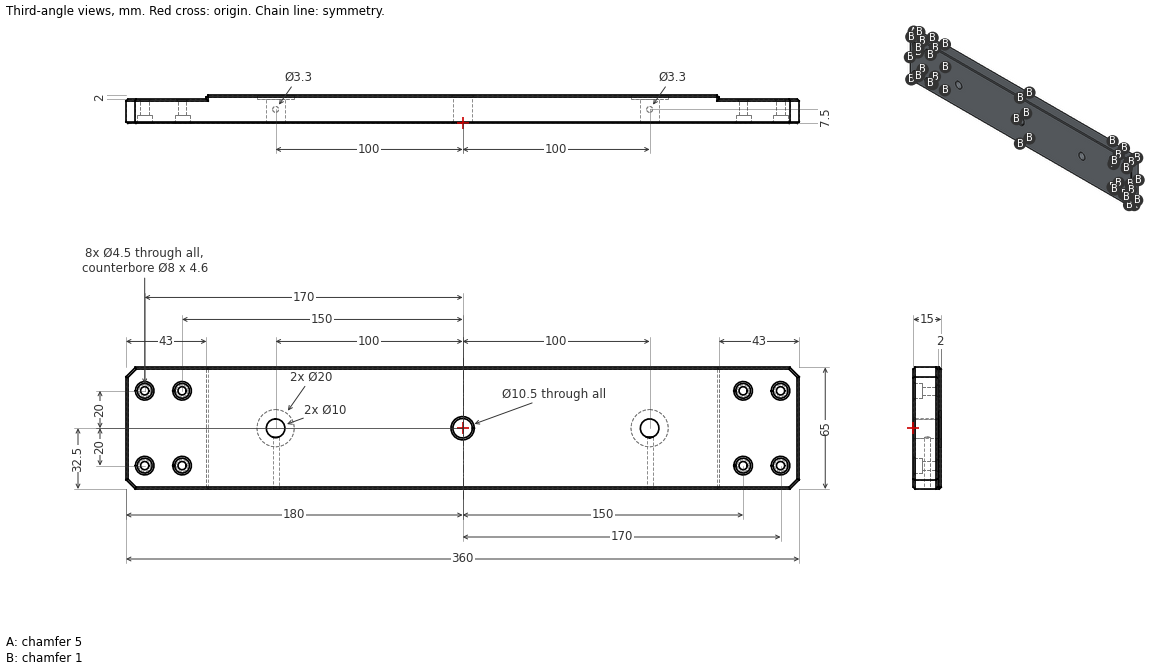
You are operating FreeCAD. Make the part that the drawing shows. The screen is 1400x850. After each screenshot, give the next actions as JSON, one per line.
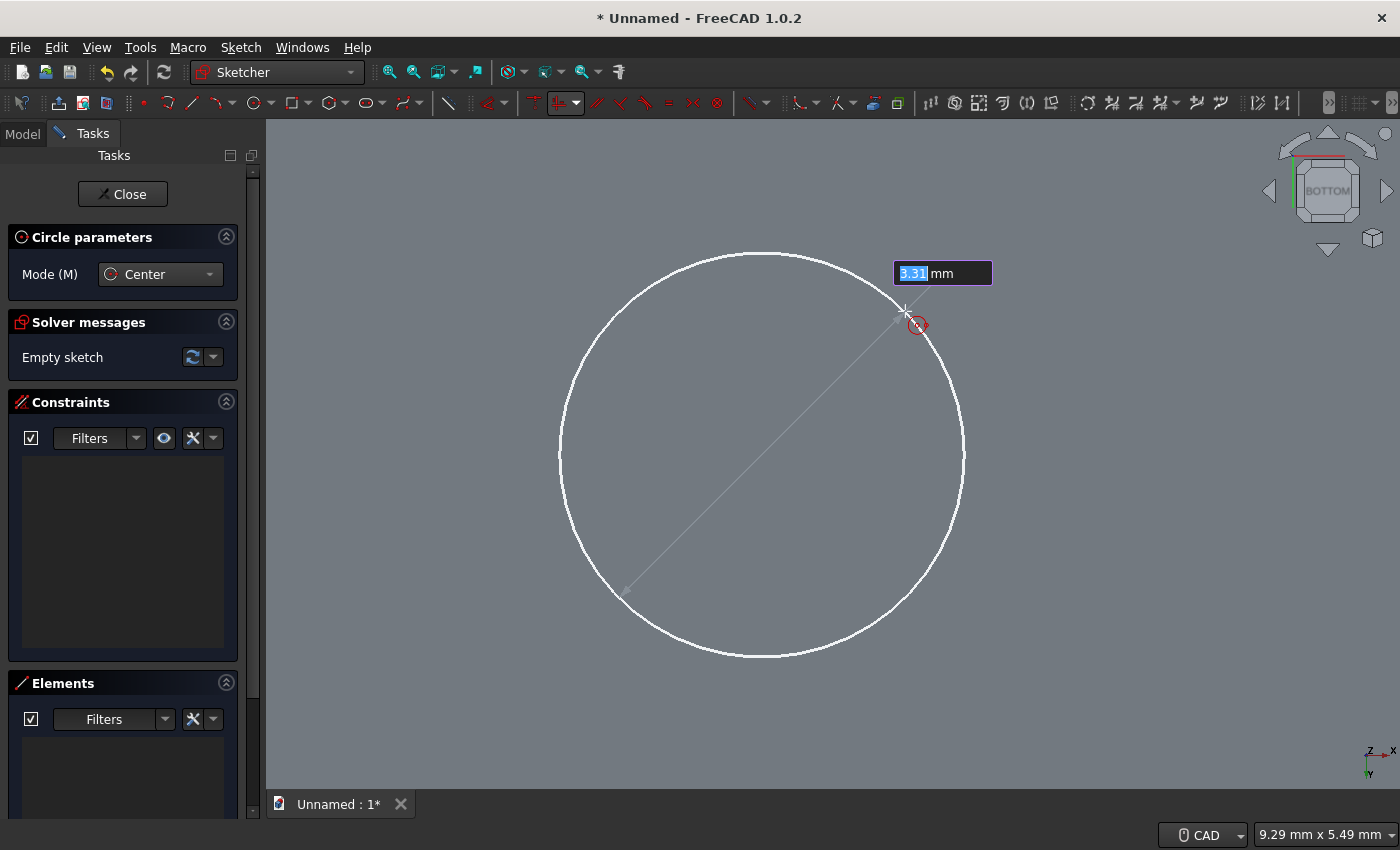
{"action": "type", "text": "3.3"}
{"action": "key", "text": "Return"}
{"action": "key", "text": "Escape"}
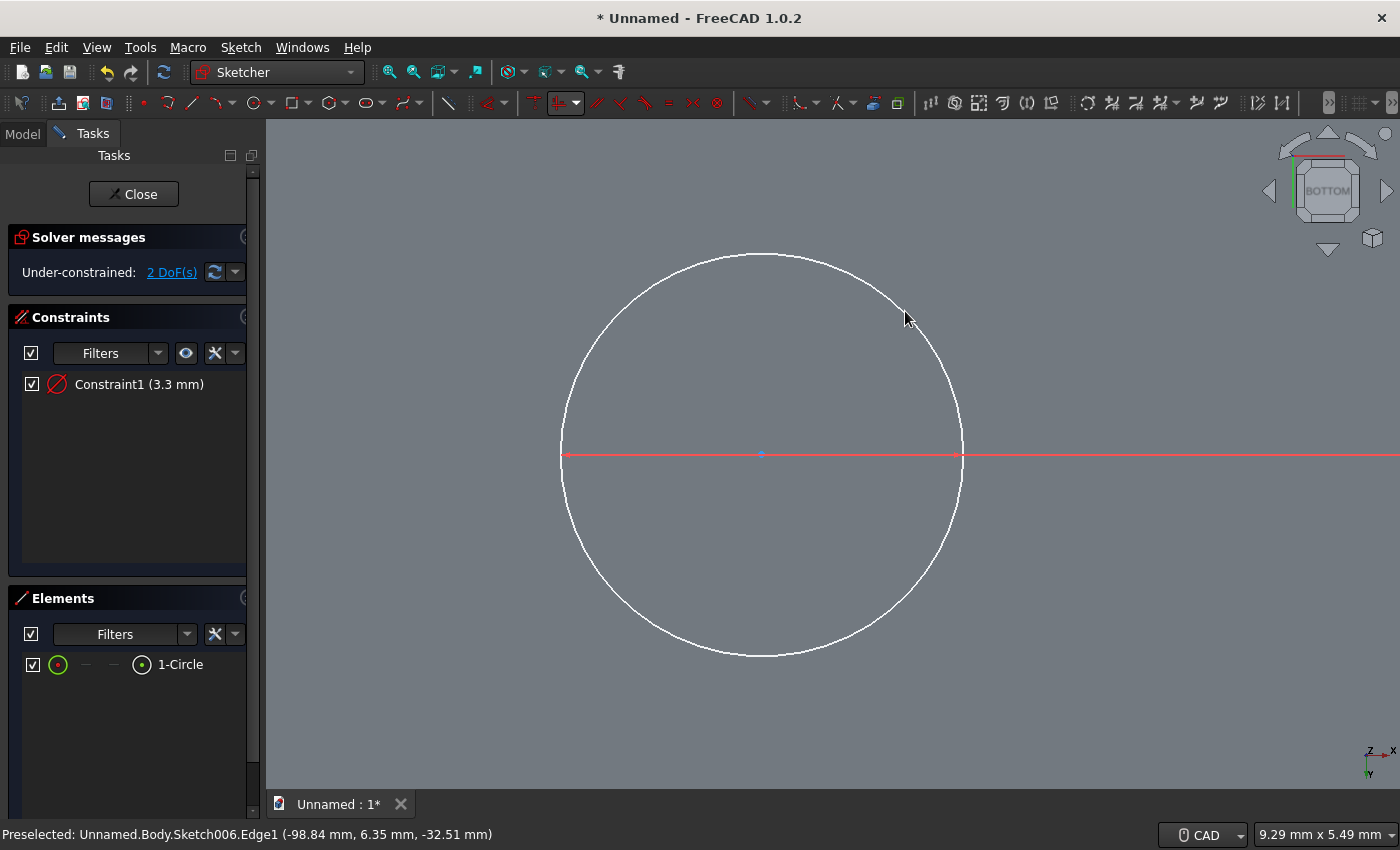
{"action": "left_click", "coordinate": [488, 104]}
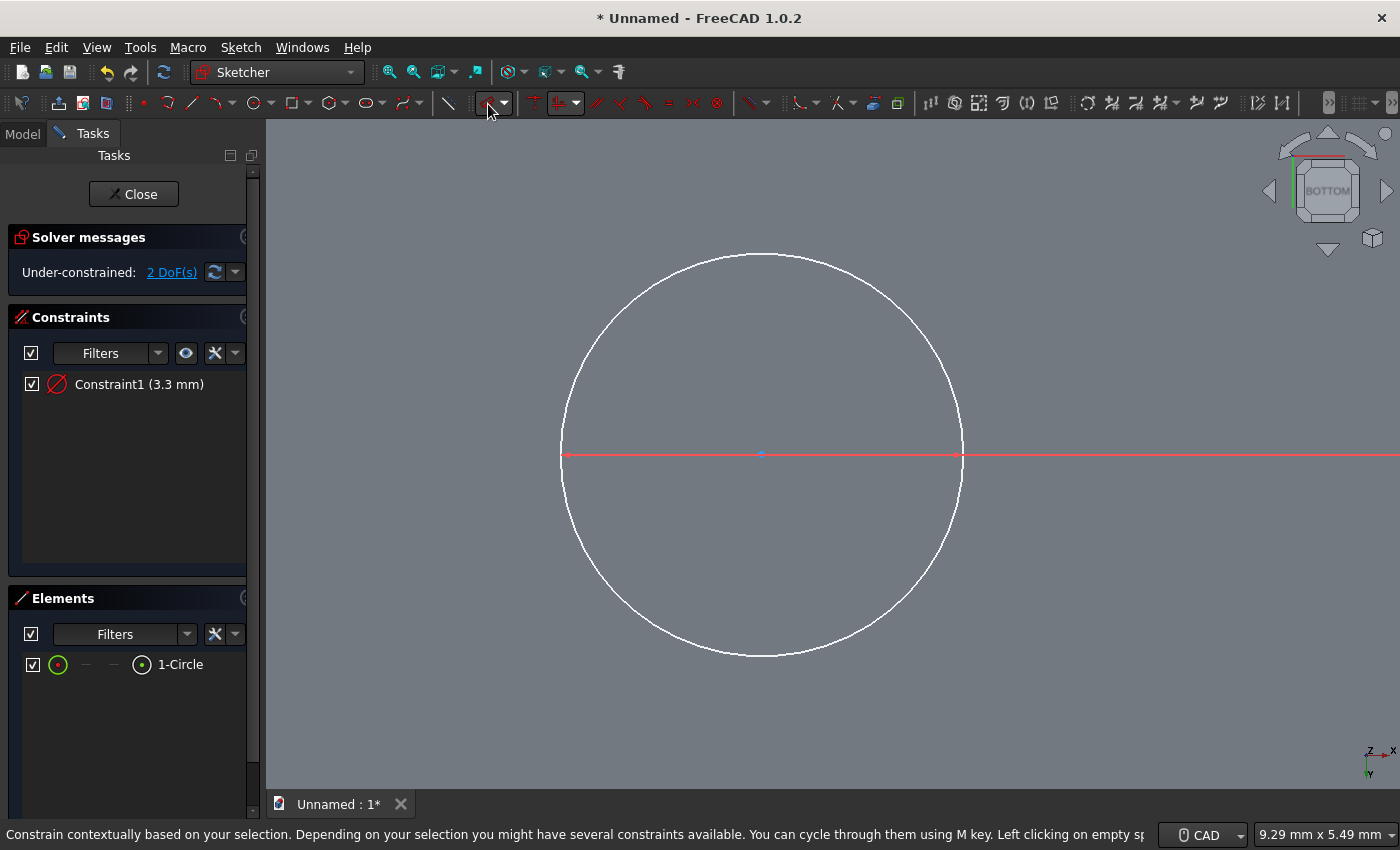
{"action": "left_click", "coordinate": [762, 455]}
{"action": "left_click", "coordinate": [998, 489]}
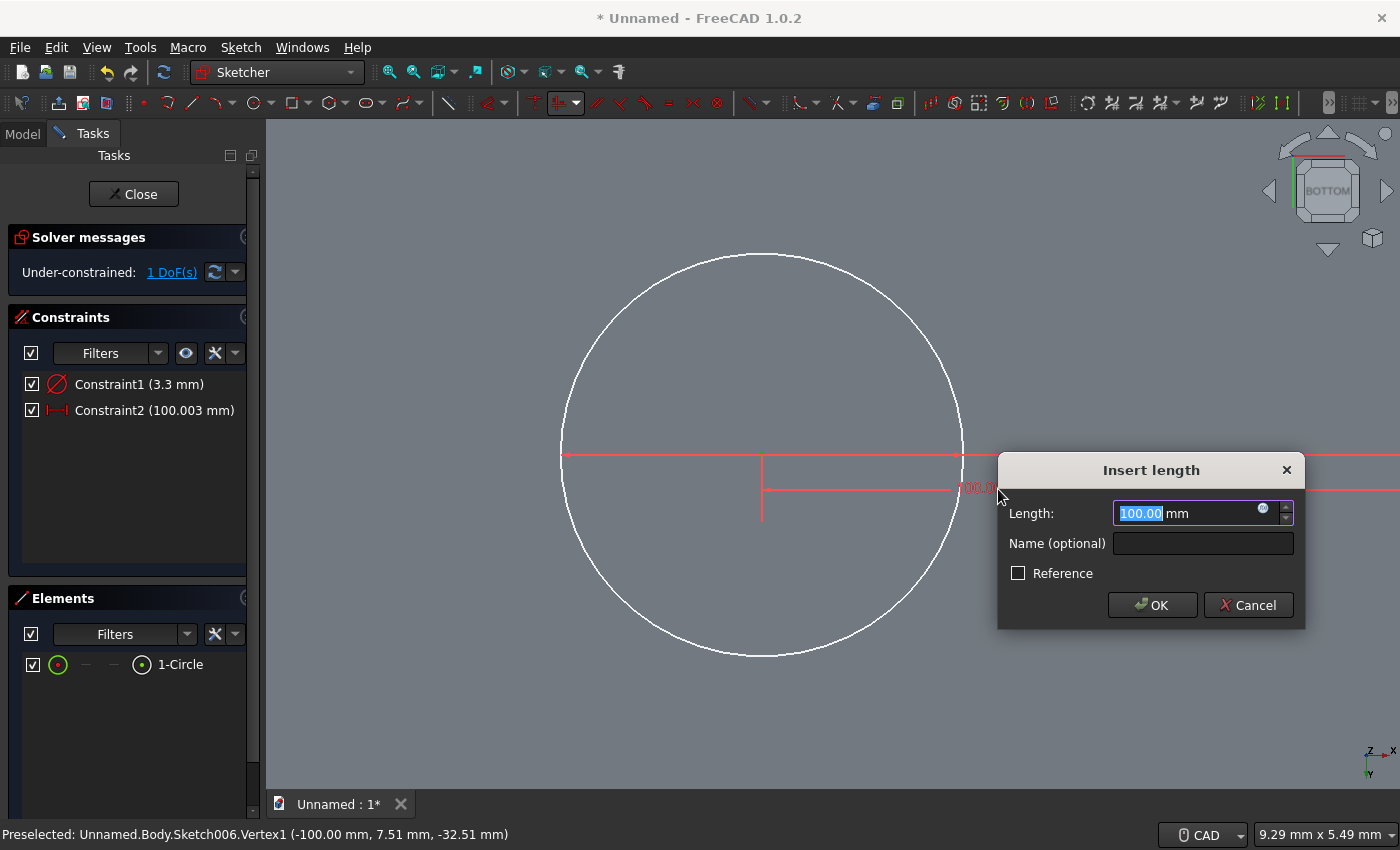
{"action": "type", "text": "100"}
{"action": "key", "text": "Return"}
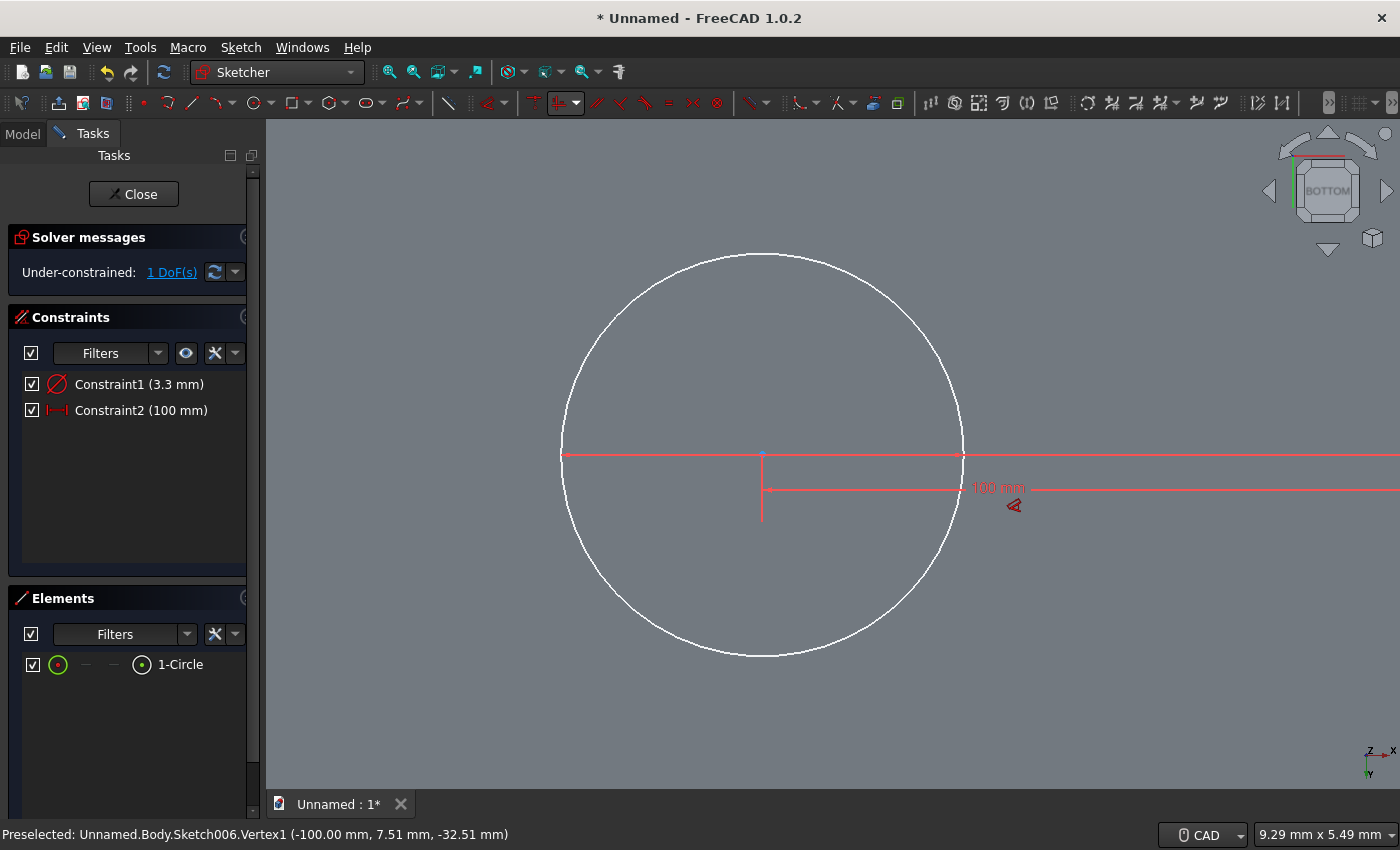
{"action": "left_click", "coordinate": [762, 455]}
{"action": "left_click", "coordinate": [728, 301]}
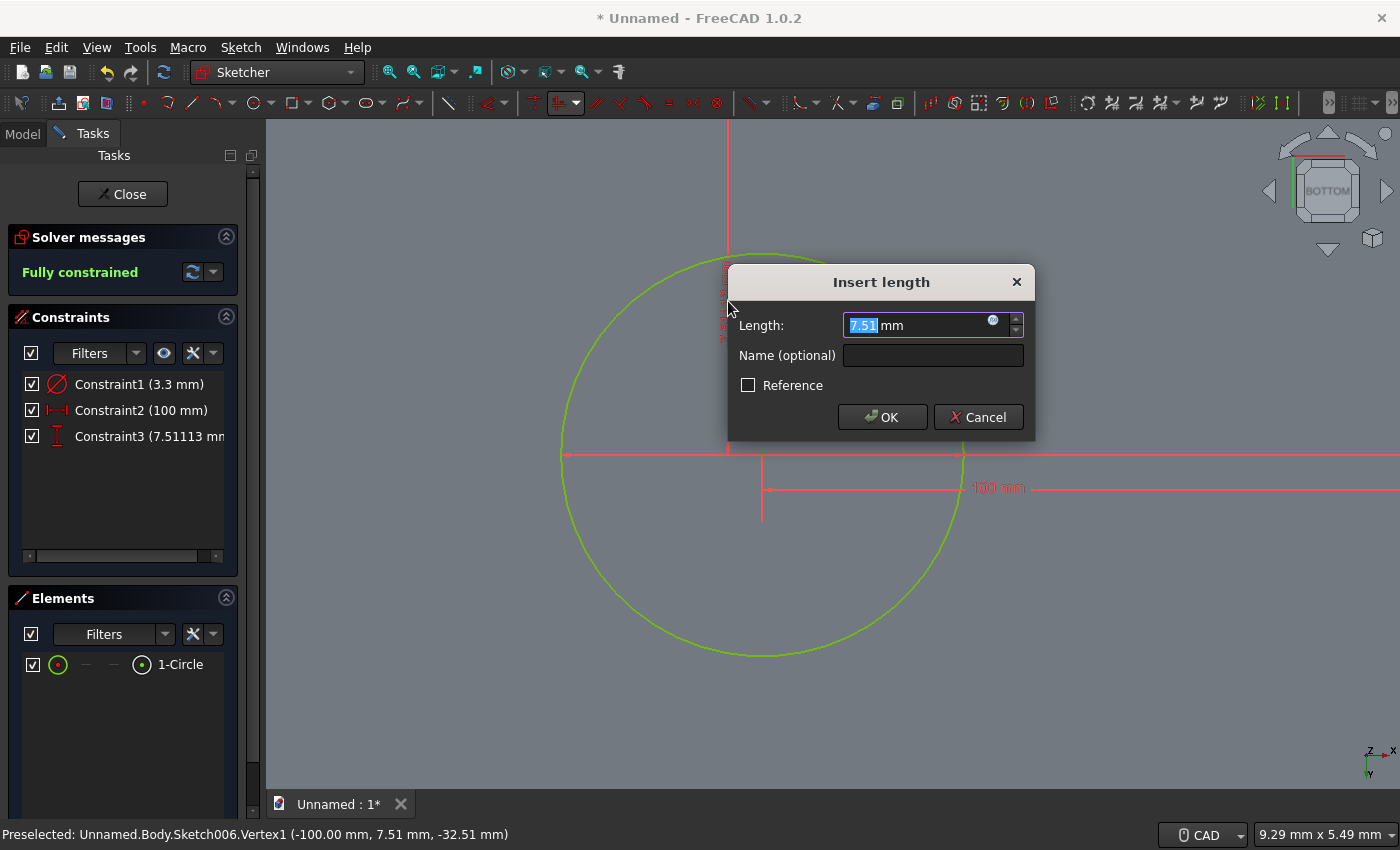
{"action": "type", "text": "7.5"}
{"action": "key", "text": "Return"}
{"action": "key", "text": "Escape"}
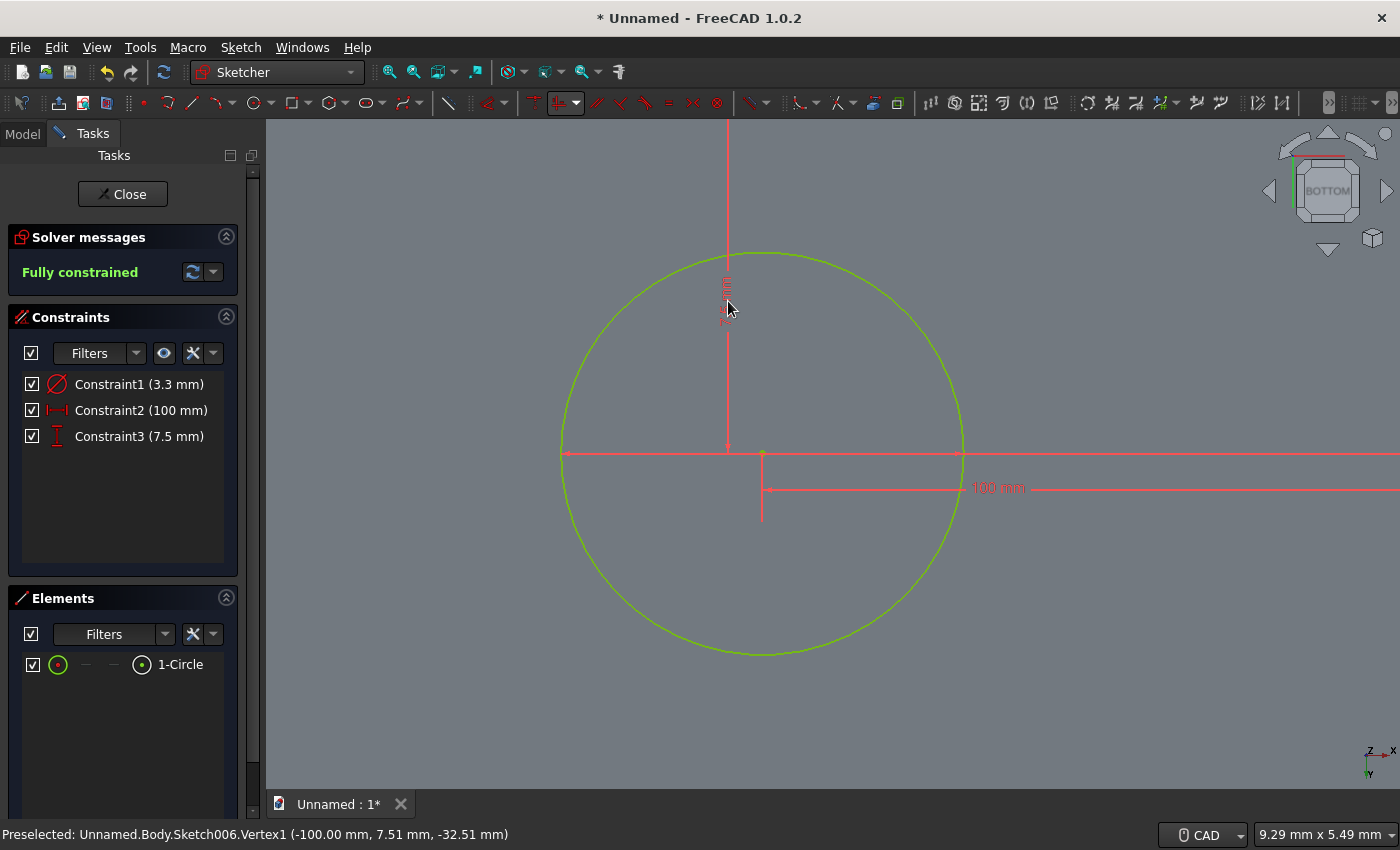
{"action": "left_click", "coordinate": [123, 194]}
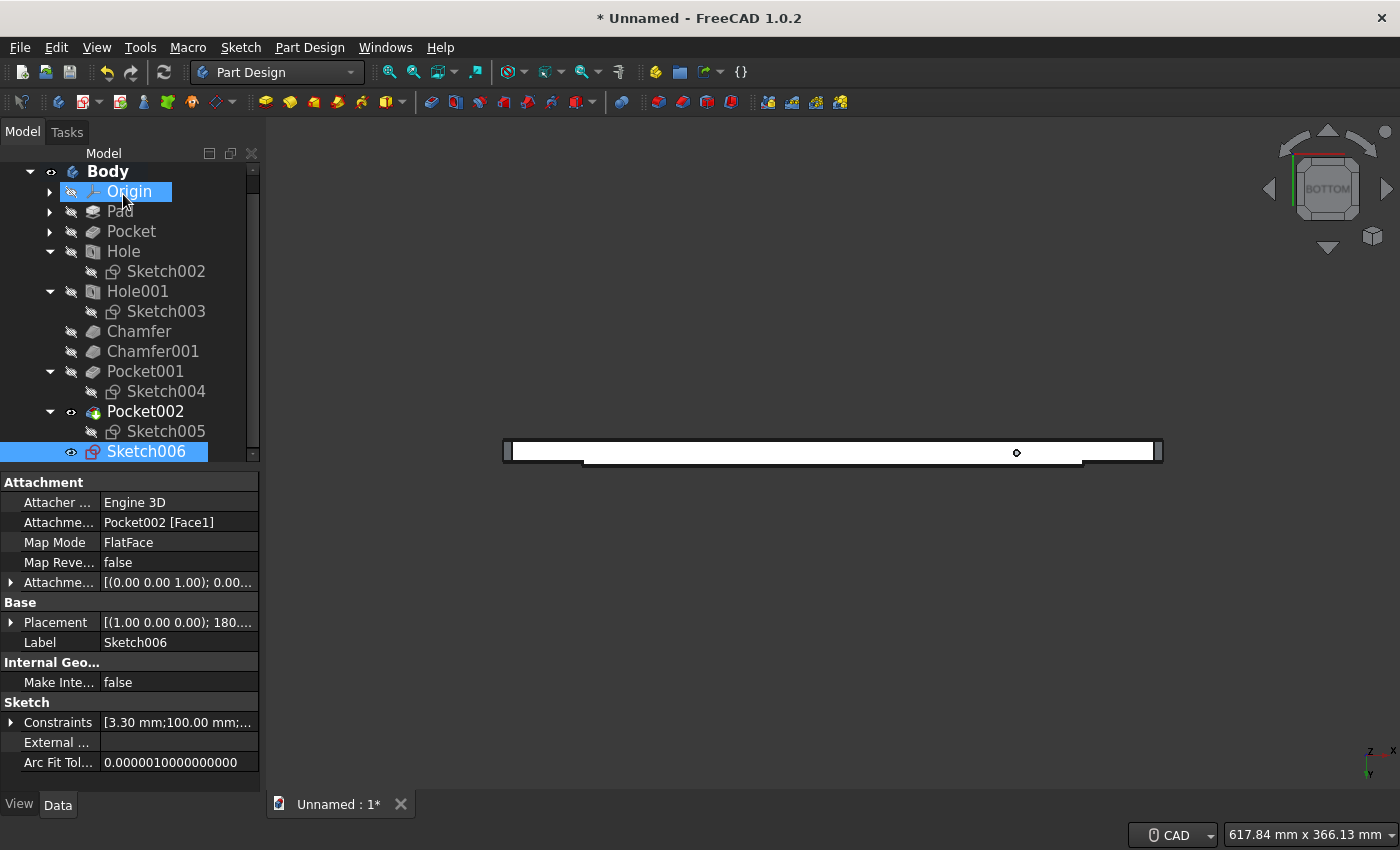
{"action": "left_click", "coordinate": [432, 102]}